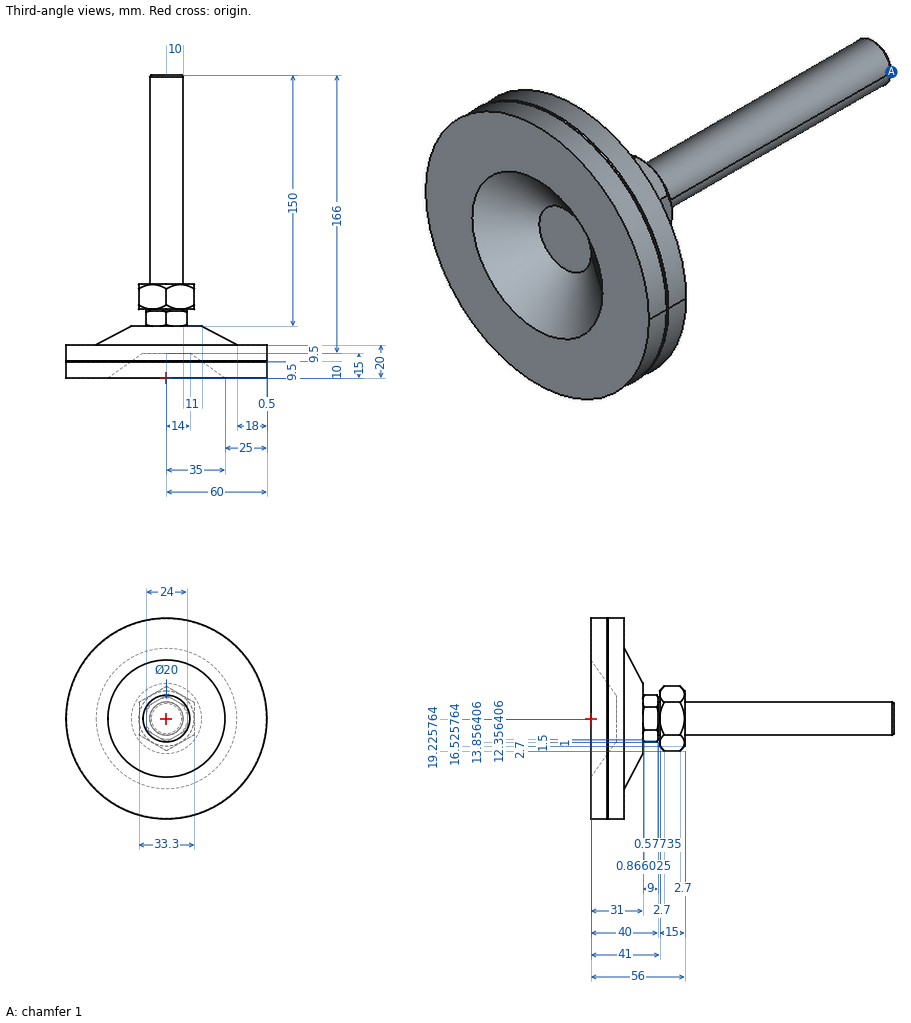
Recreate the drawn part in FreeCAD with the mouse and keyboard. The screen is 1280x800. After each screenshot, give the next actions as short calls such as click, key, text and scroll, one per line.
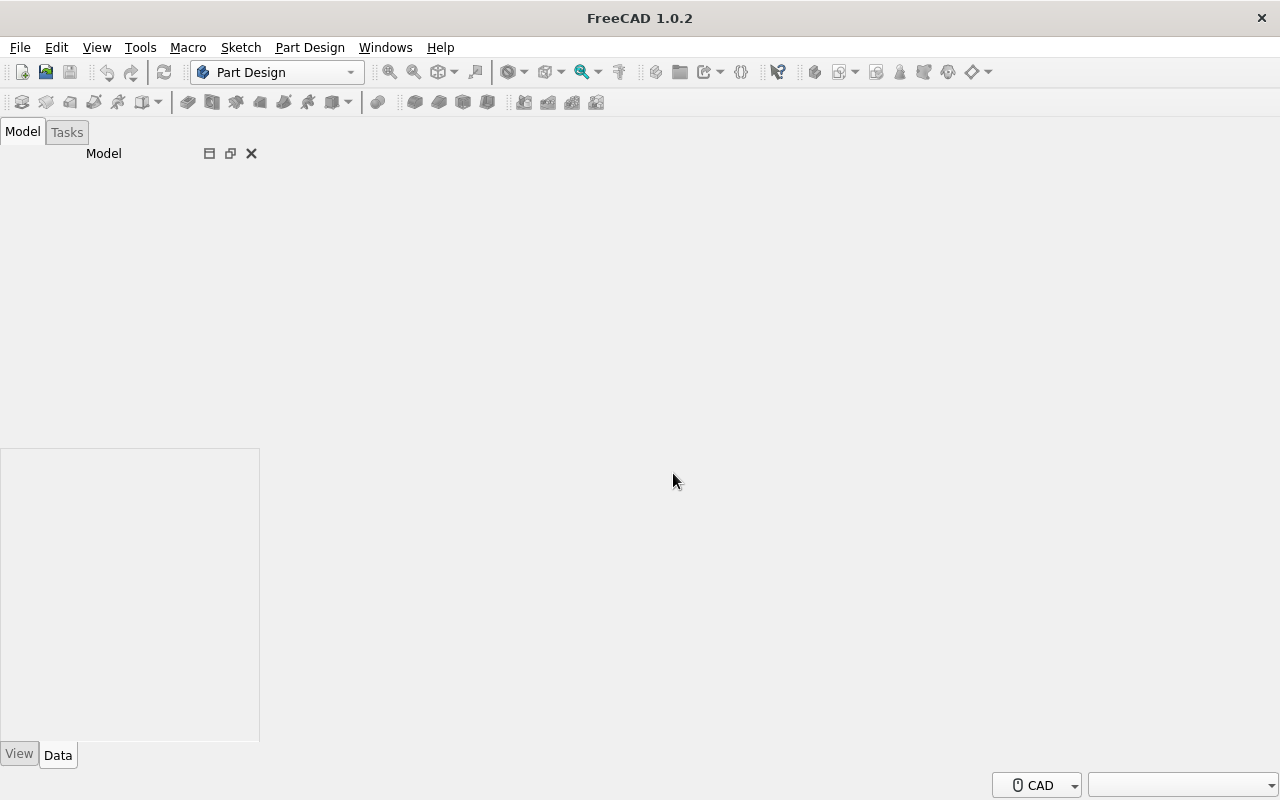
click(22, 72)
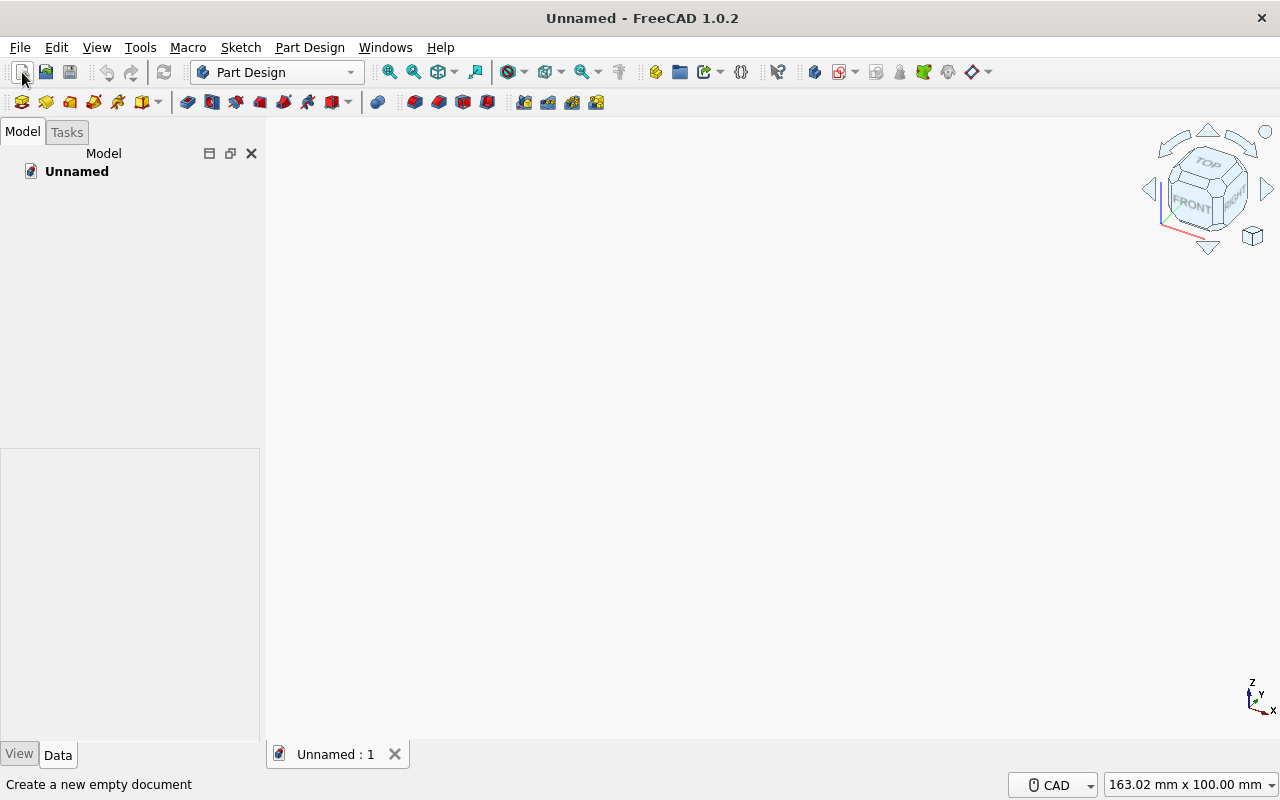
click(840, 72)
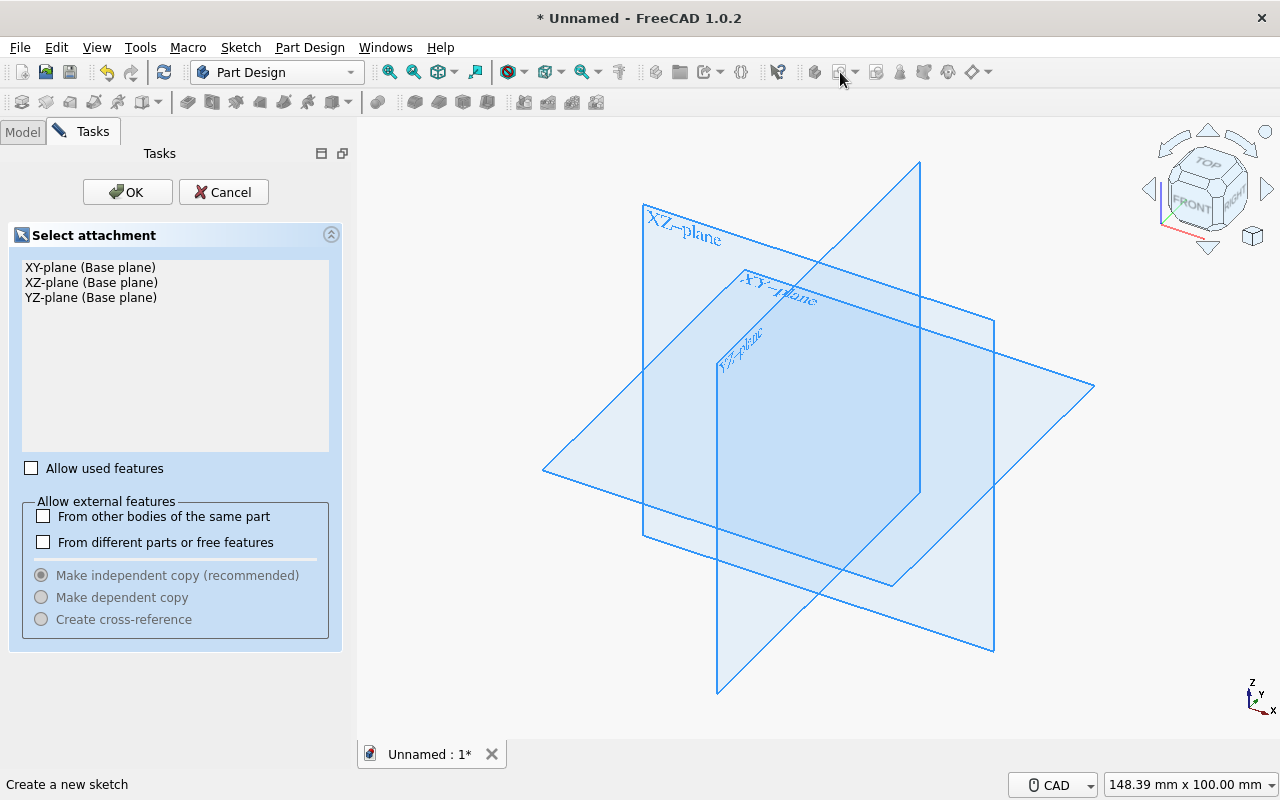
click(82, 268)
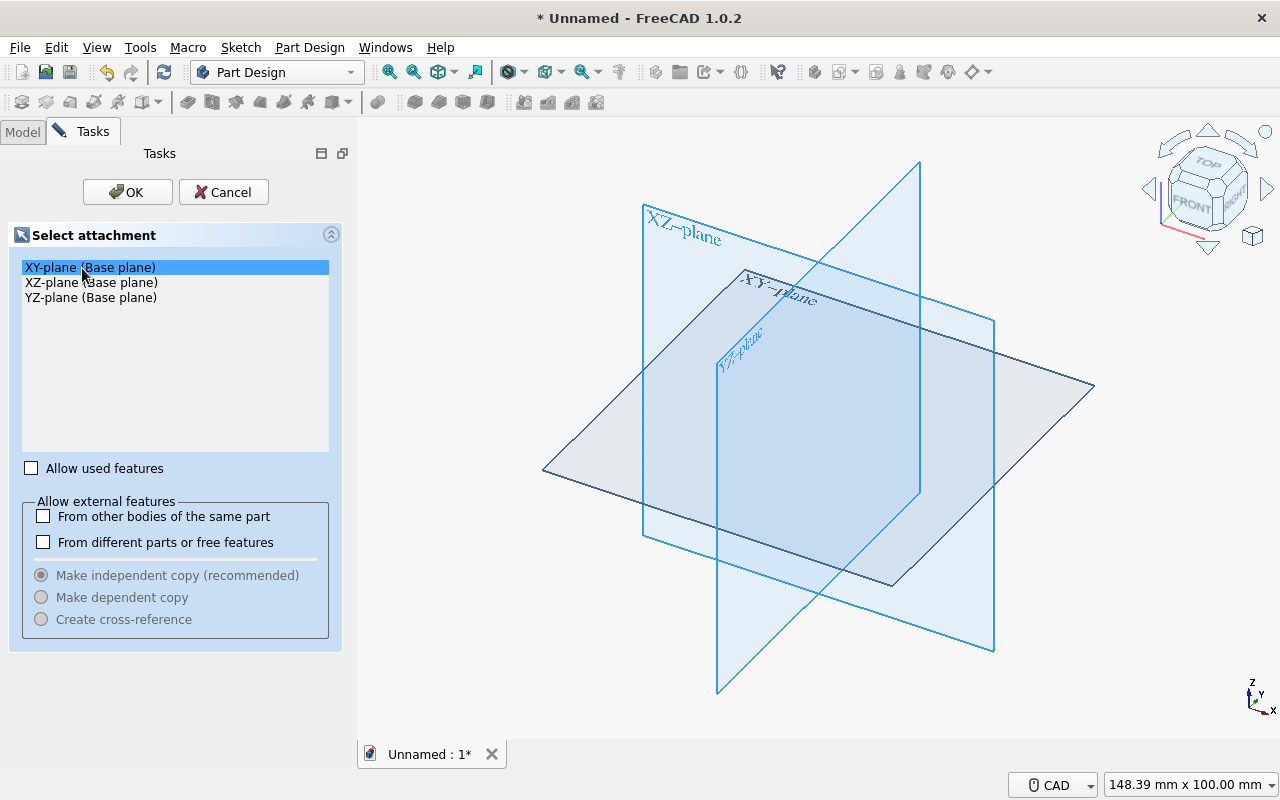
click(128, 192)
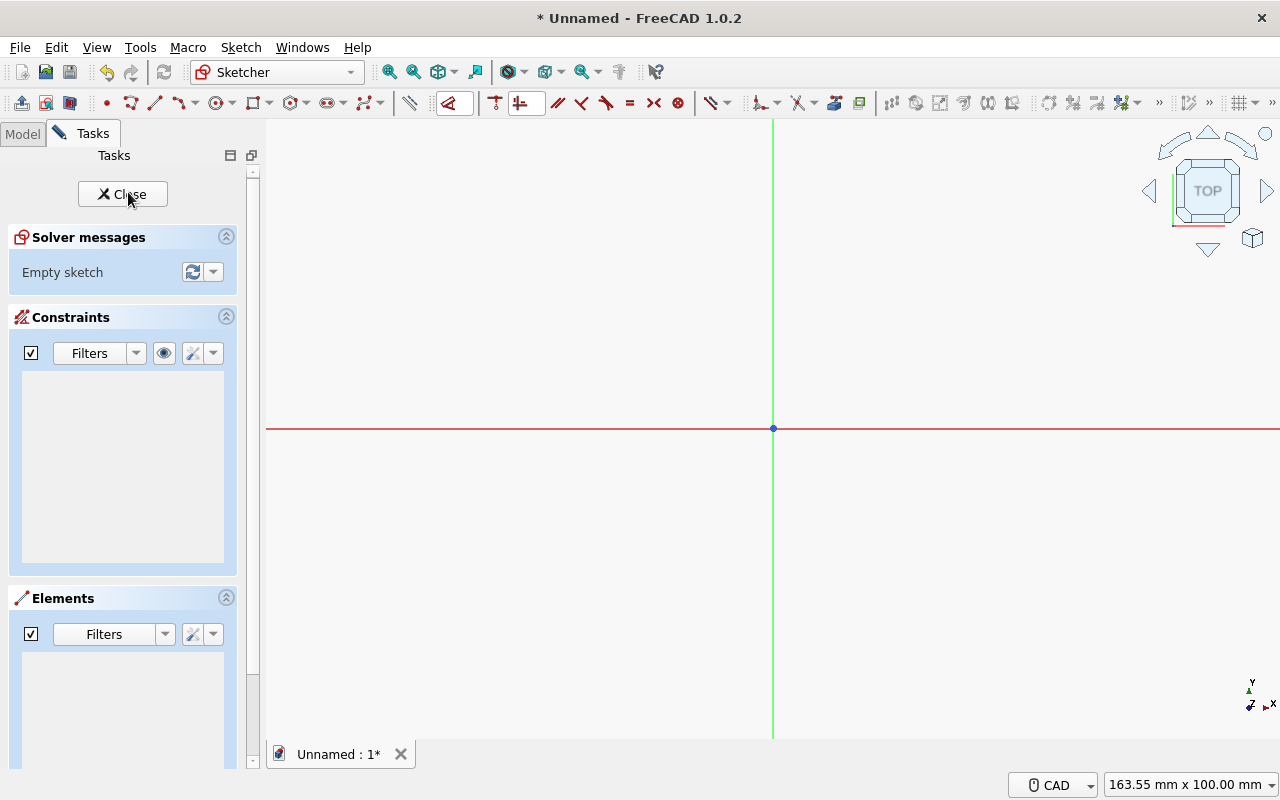
scroll(556, 711, down, 5)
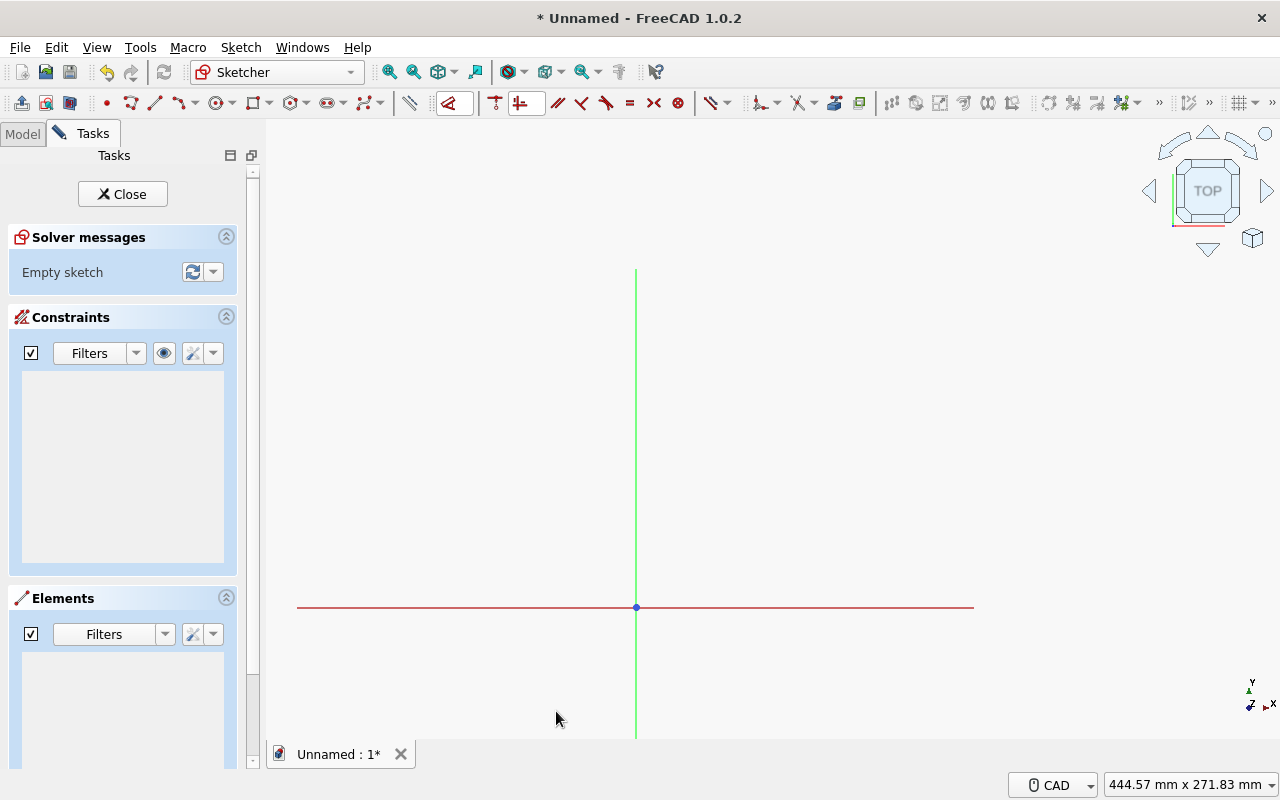
click(132, 104)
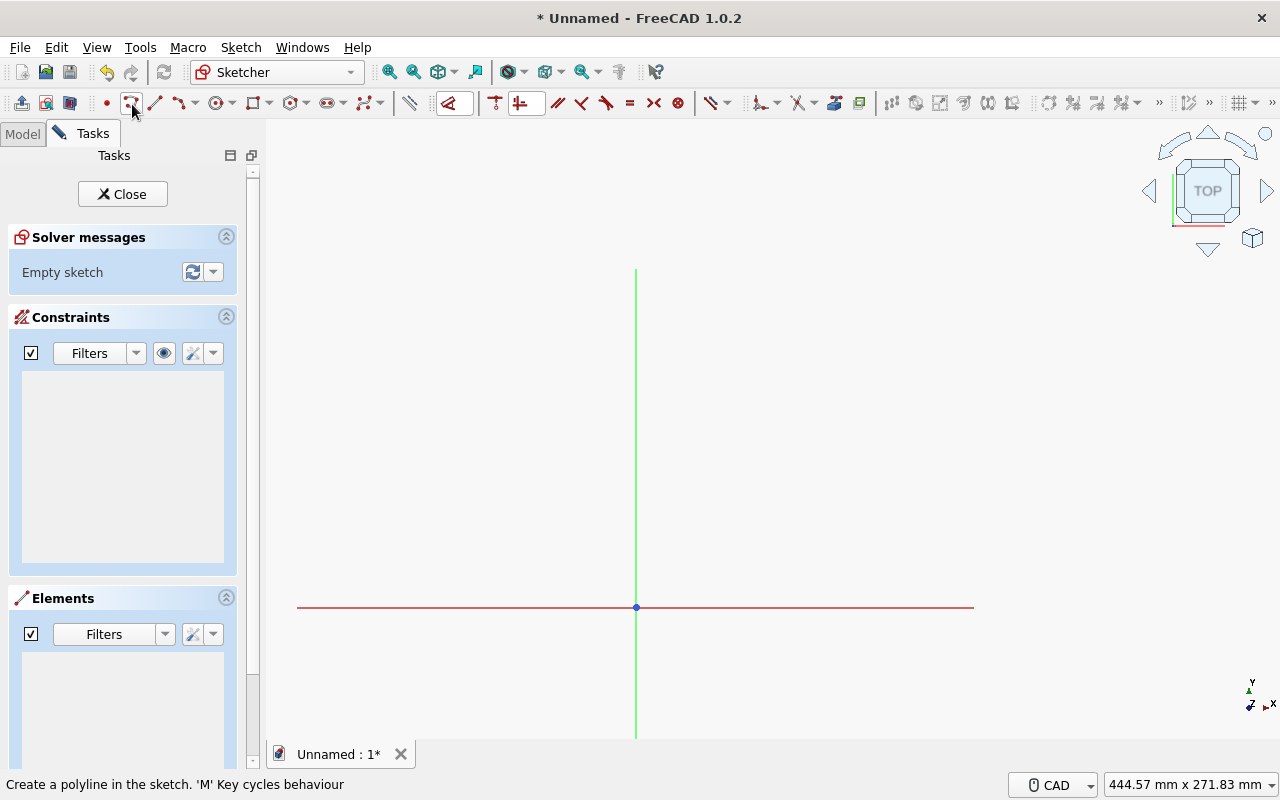
click(636, 574)
click(668, 574)
click(716, 608)
click(773, 599)
click(773, 586)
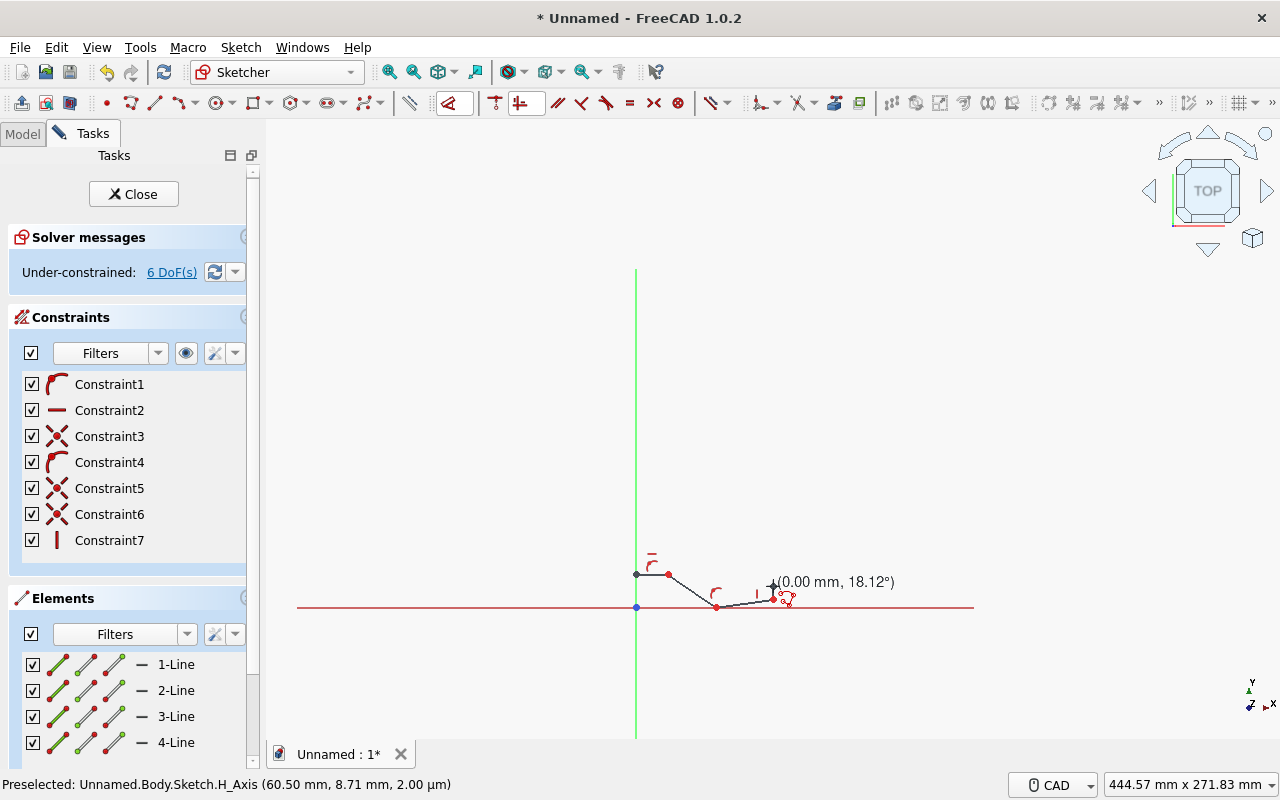
scroll(772, 585, up, 12)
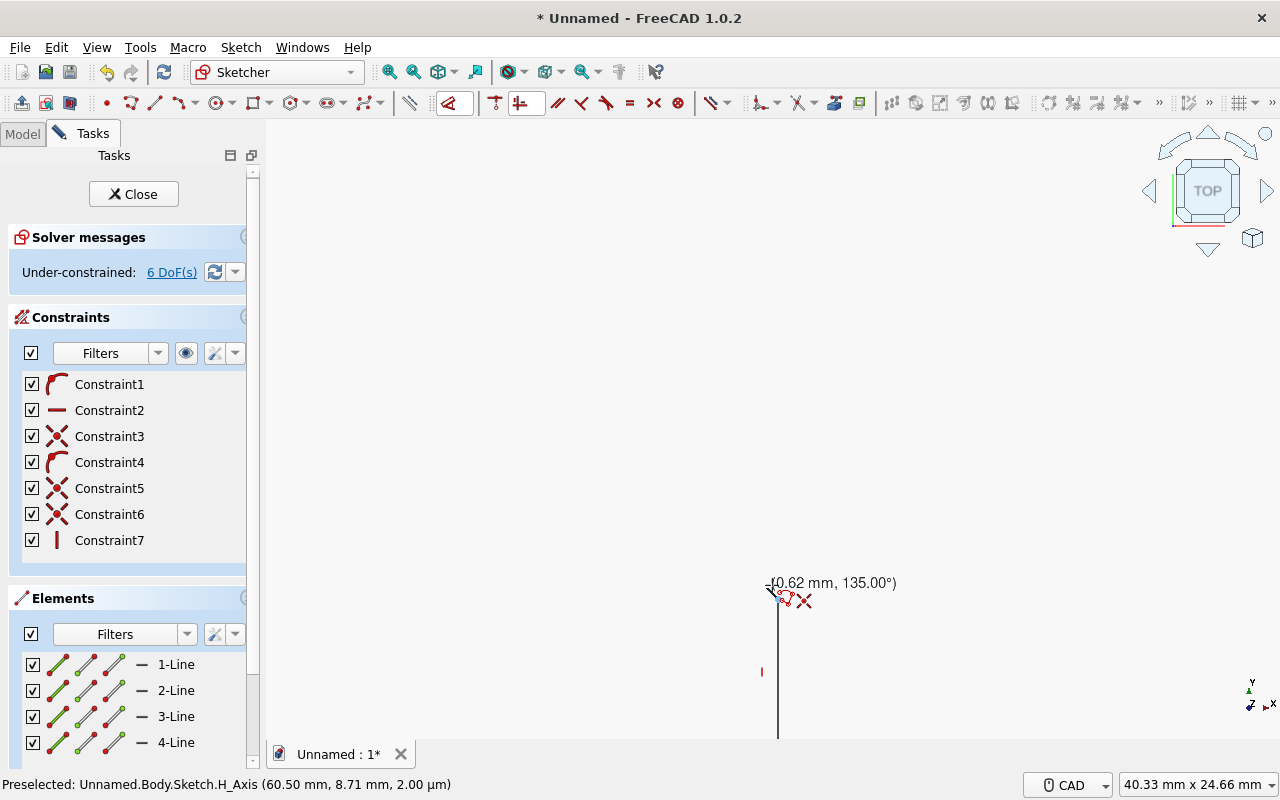
click(764, 578)
click(776, 565)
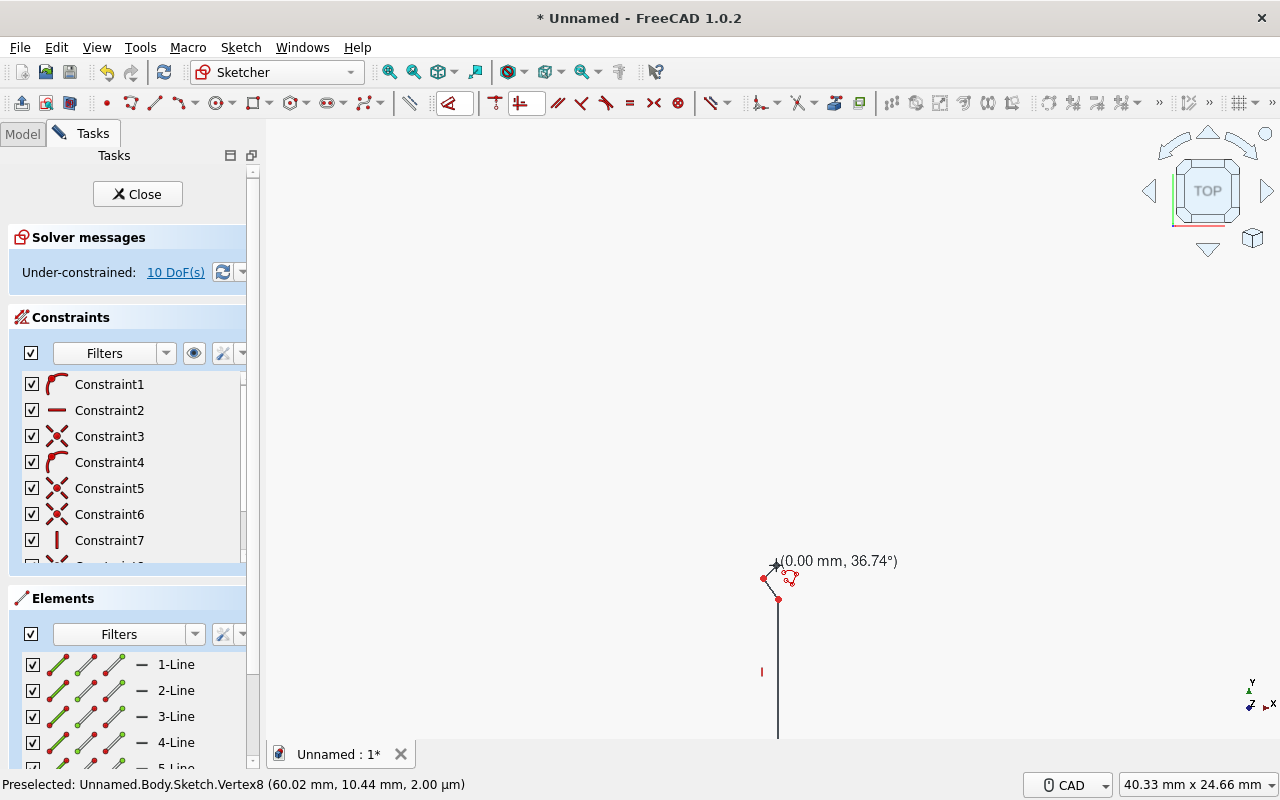
scroll(773, 616, down, 12)